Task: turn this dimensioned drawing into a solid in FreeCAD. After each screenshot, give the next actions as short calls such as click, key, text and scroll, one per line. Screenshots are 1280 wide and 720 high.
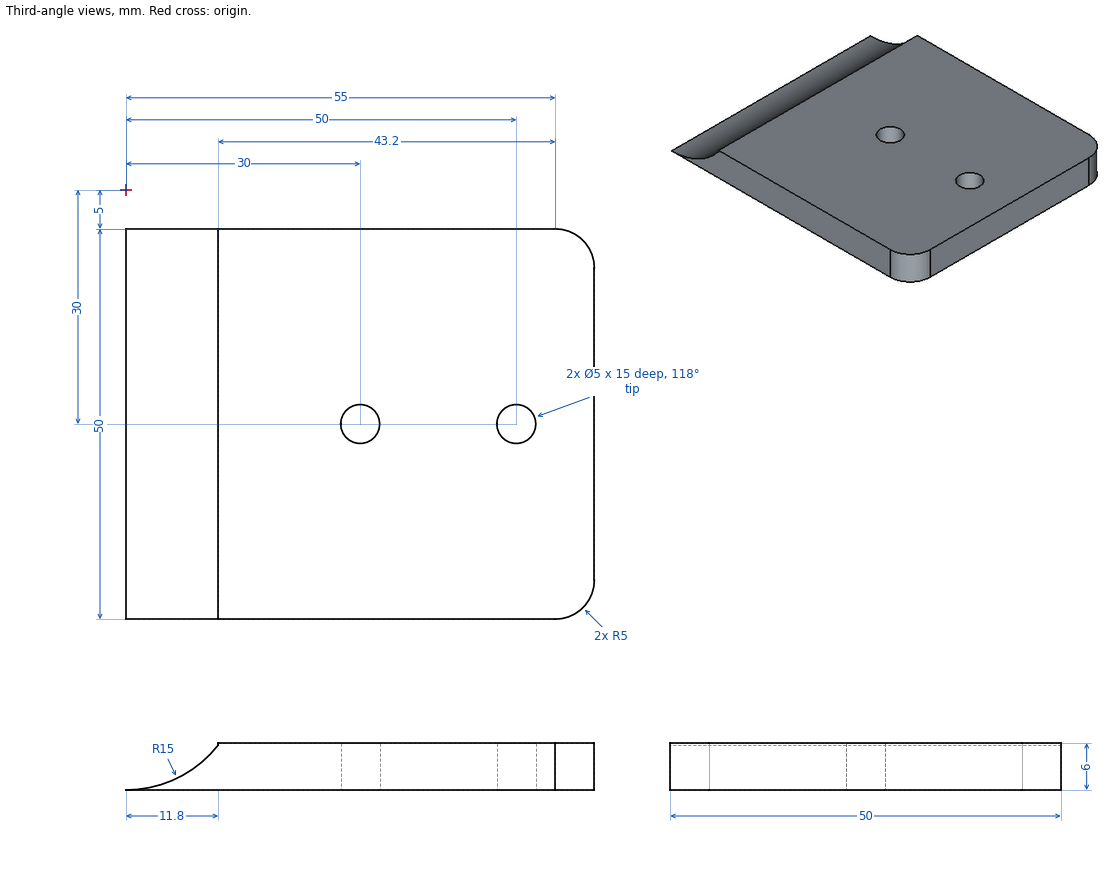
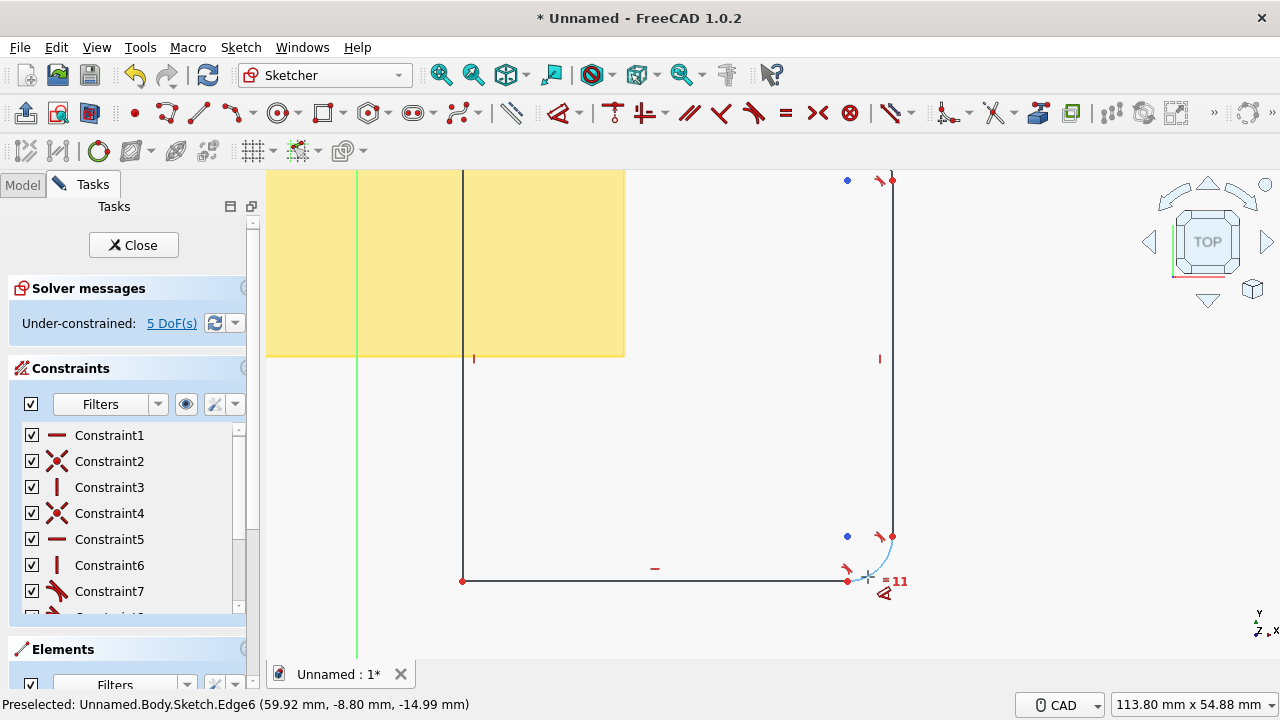
click(868, 576)
click(883, 604)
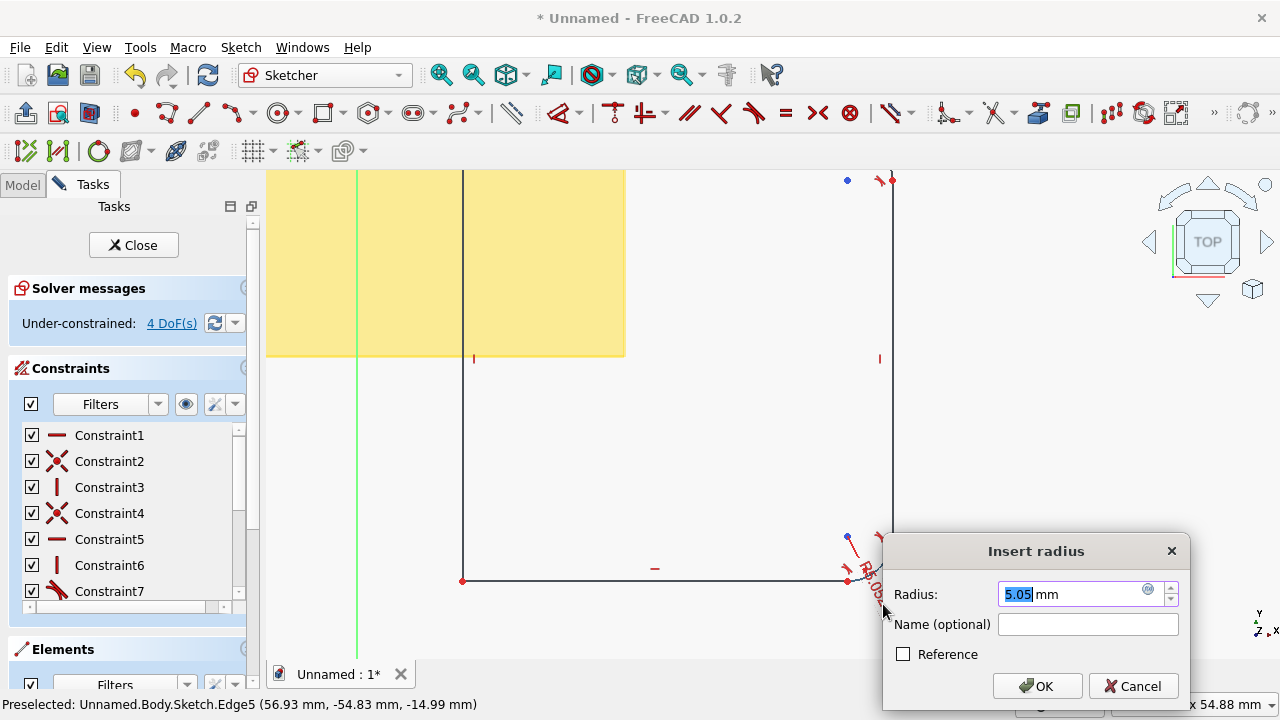
text(5)
key(Return)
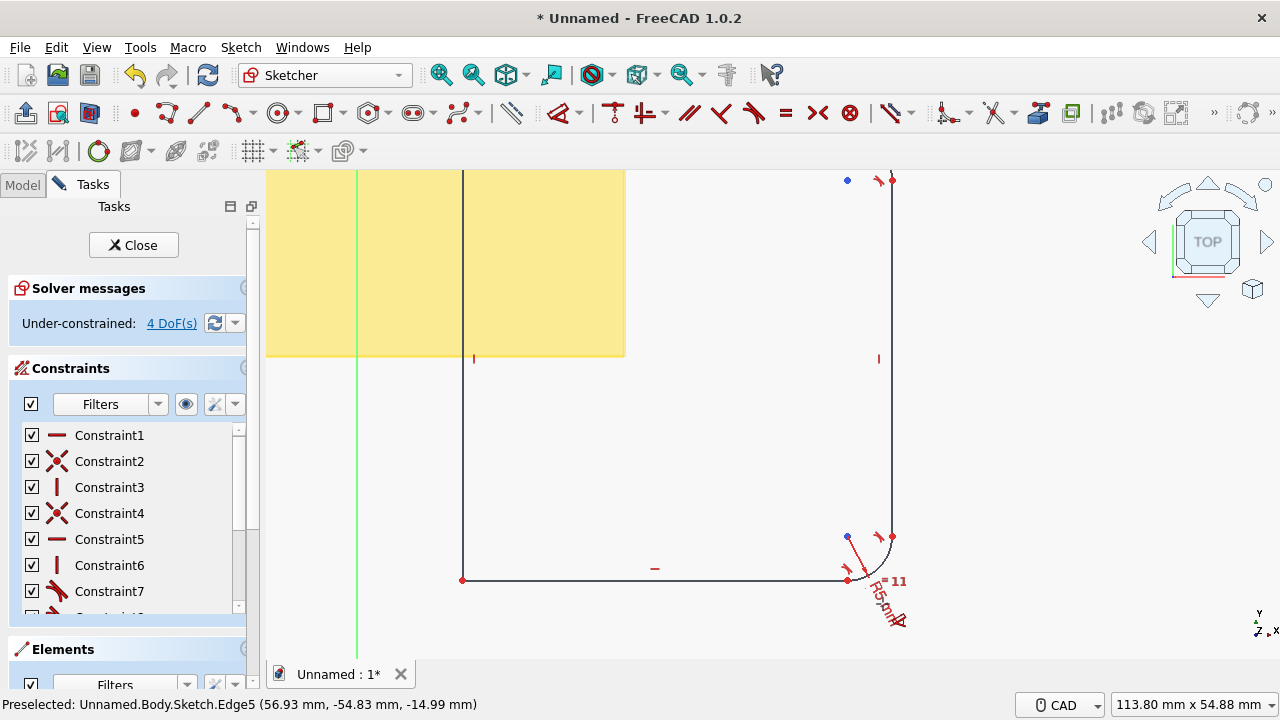
click(463, 269)
click(429, 389)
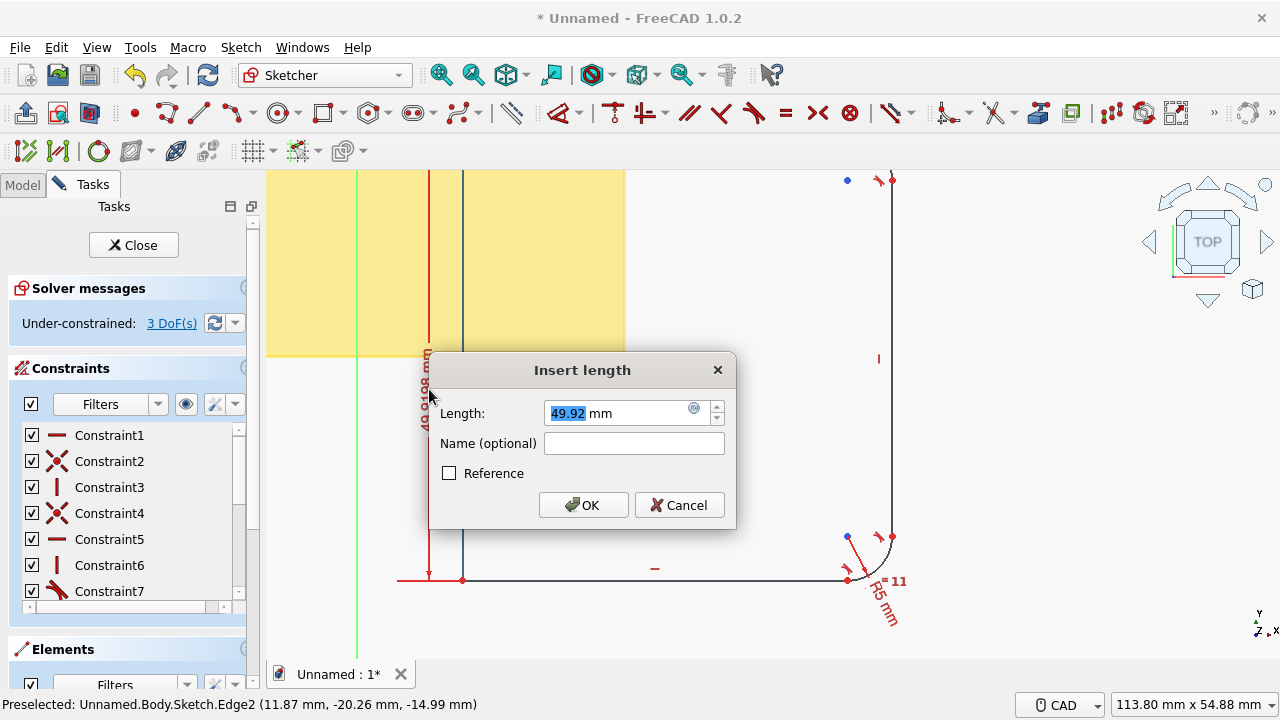
text(50)
key(Return)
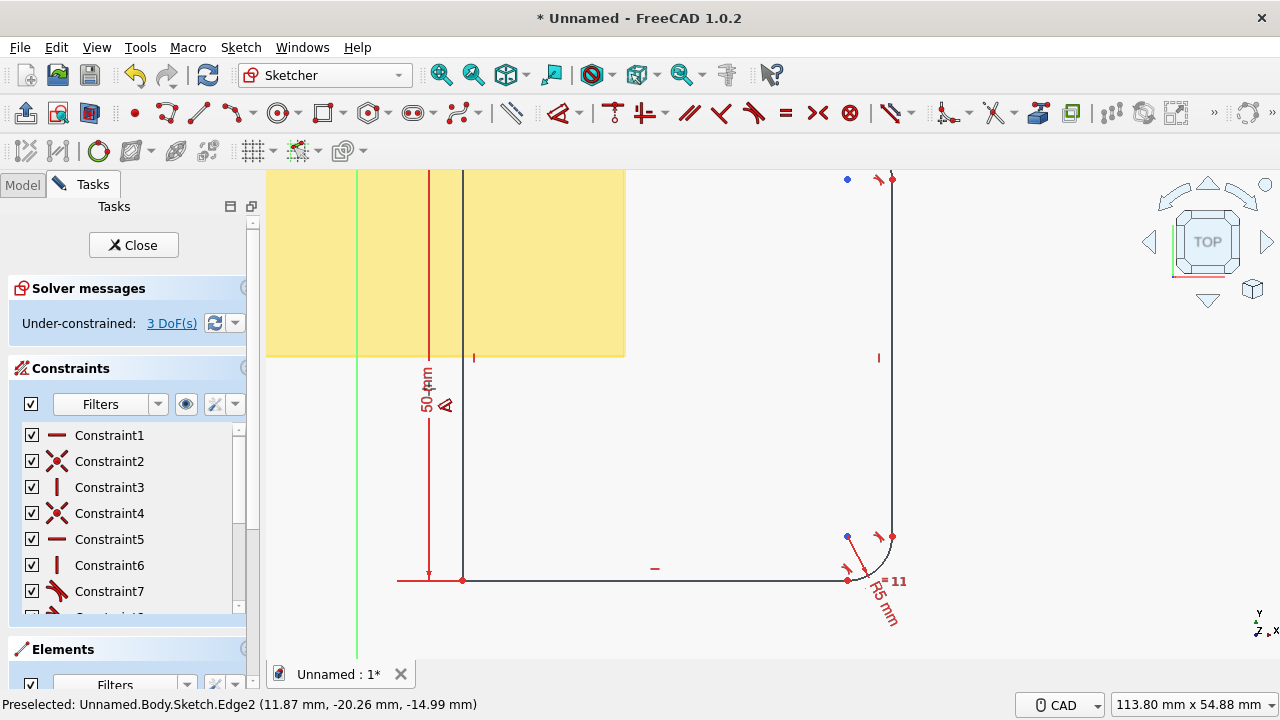
scroll(868, 577, down, 2)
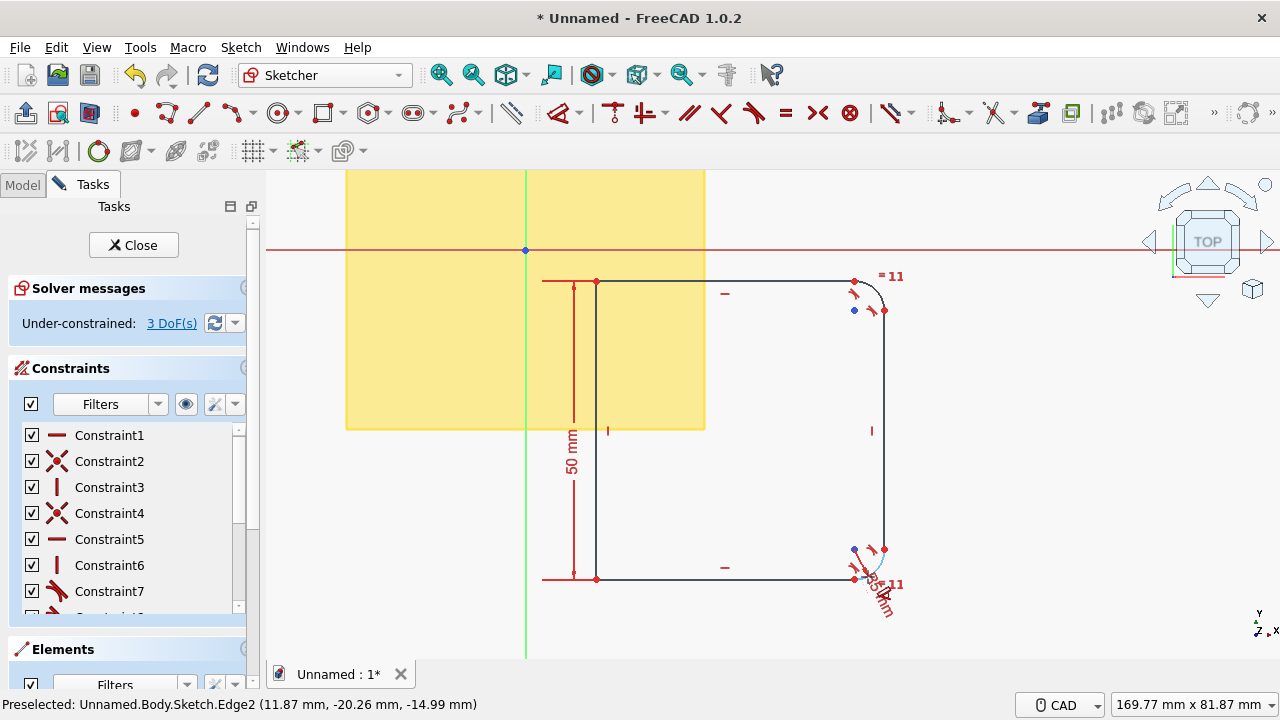
scroll(854, 281, up, 2)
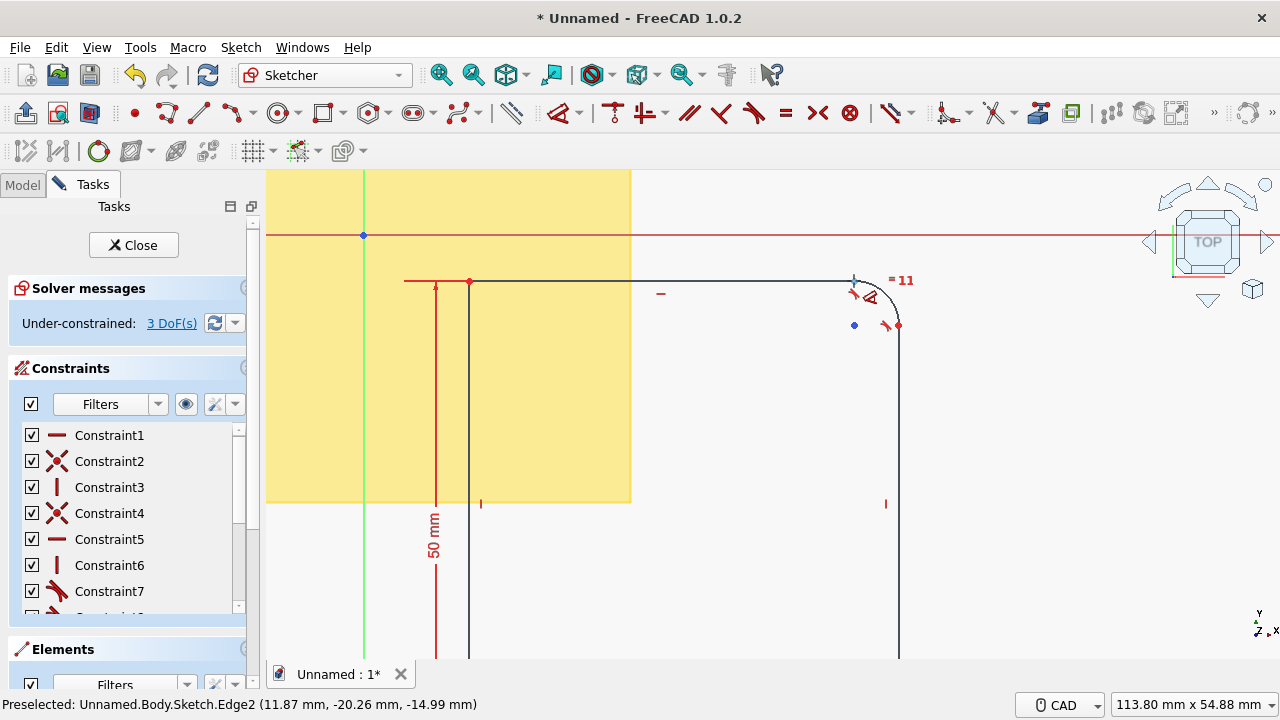
click(854, 281)
click(330, 258)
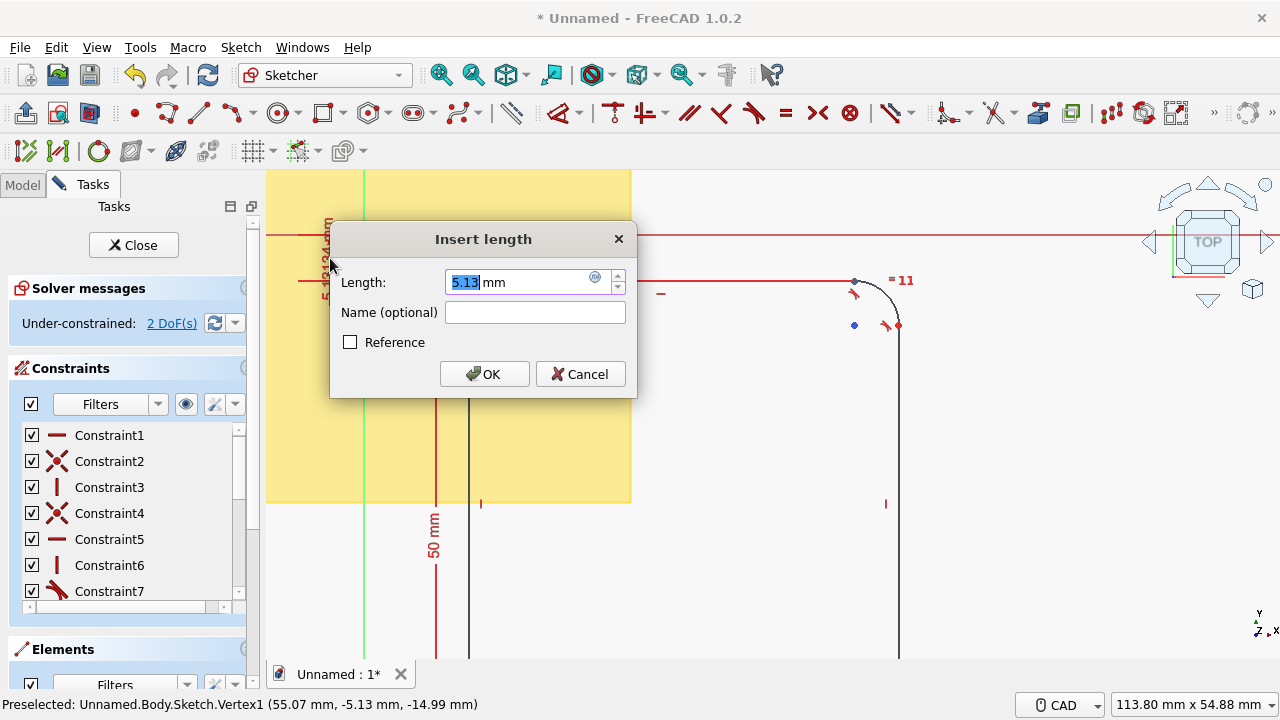
text(5)
key(Return)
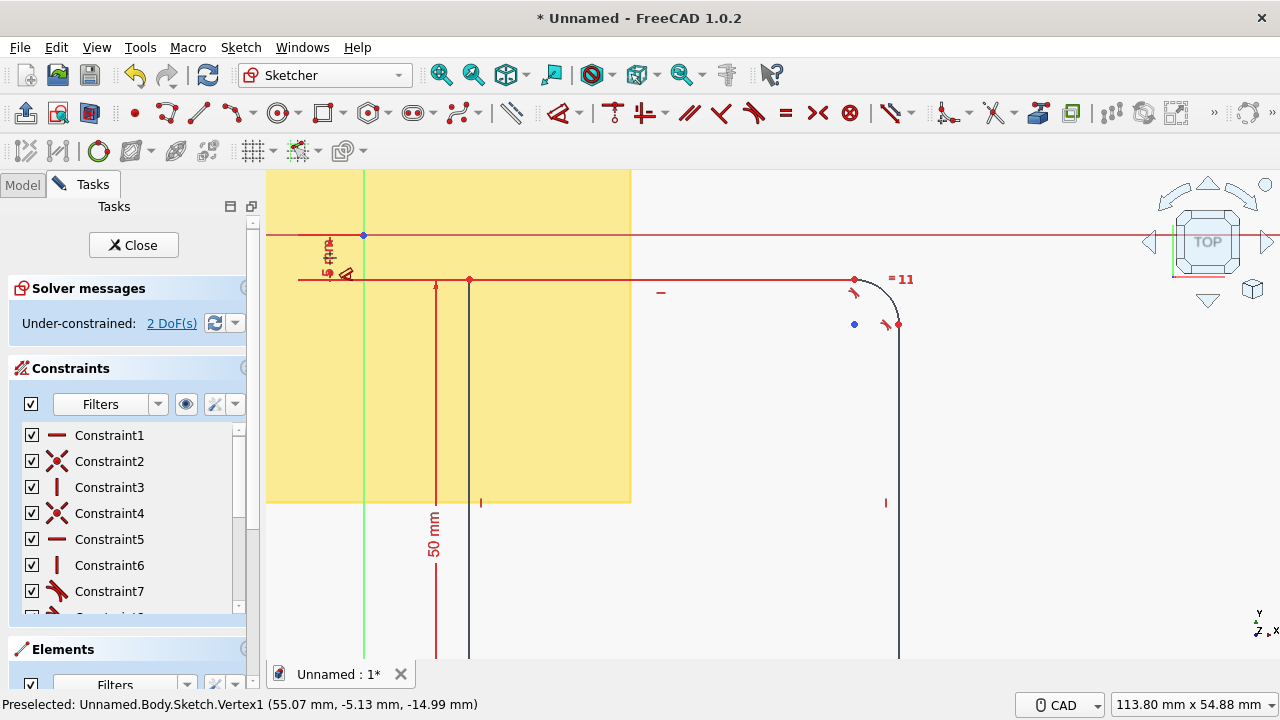
click(854, 280)
click(609, 201)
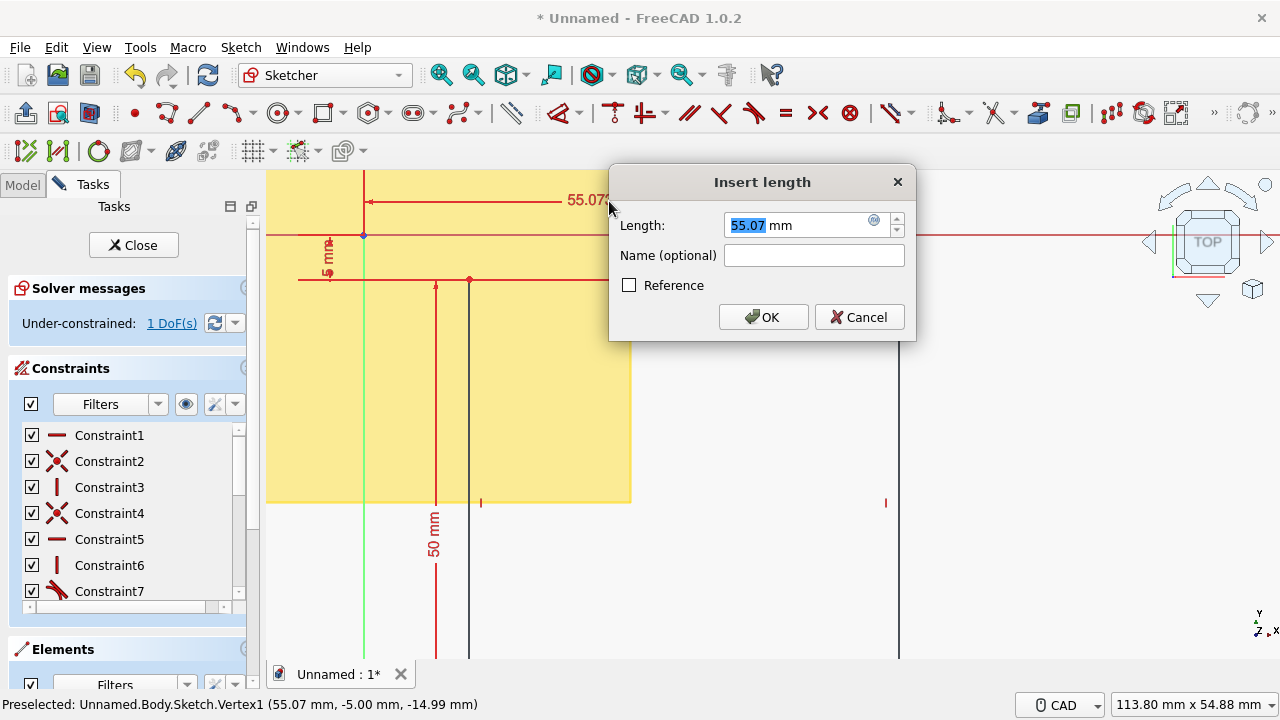
text(55)
key(Return)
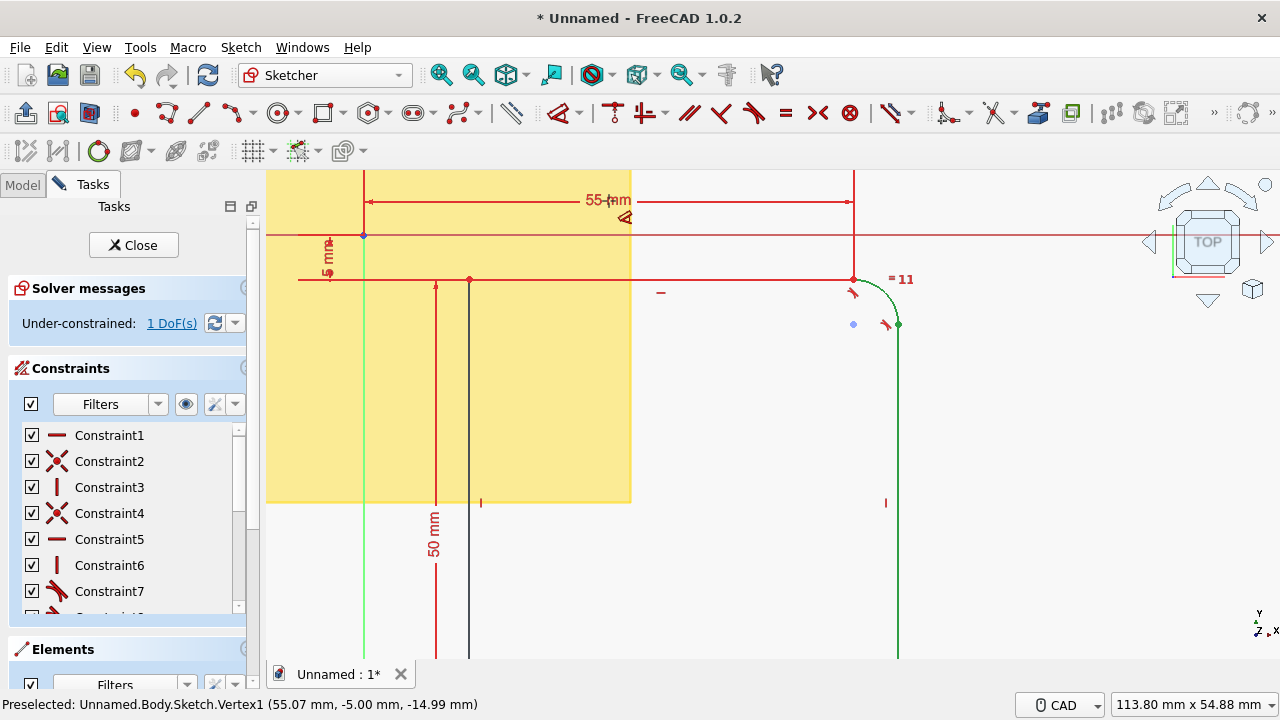
click(738, 280)
click(662, 314)